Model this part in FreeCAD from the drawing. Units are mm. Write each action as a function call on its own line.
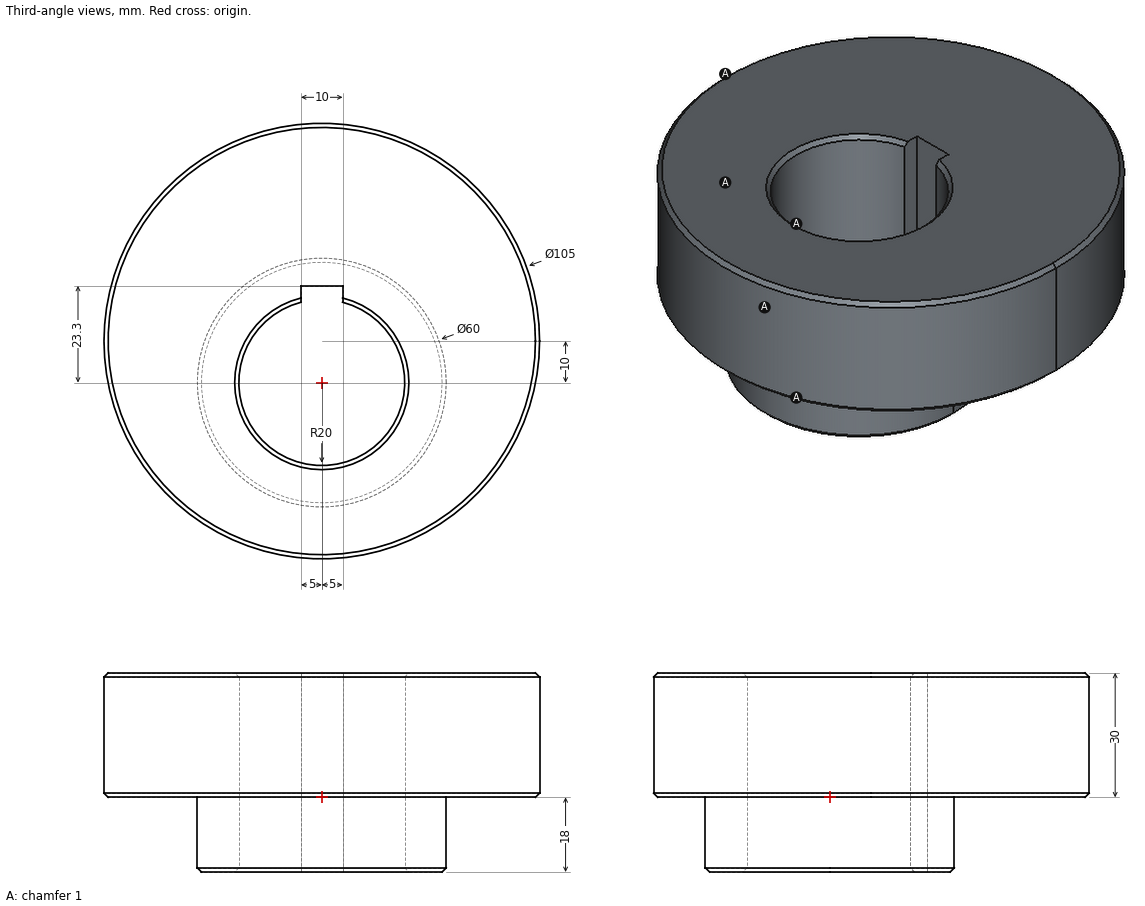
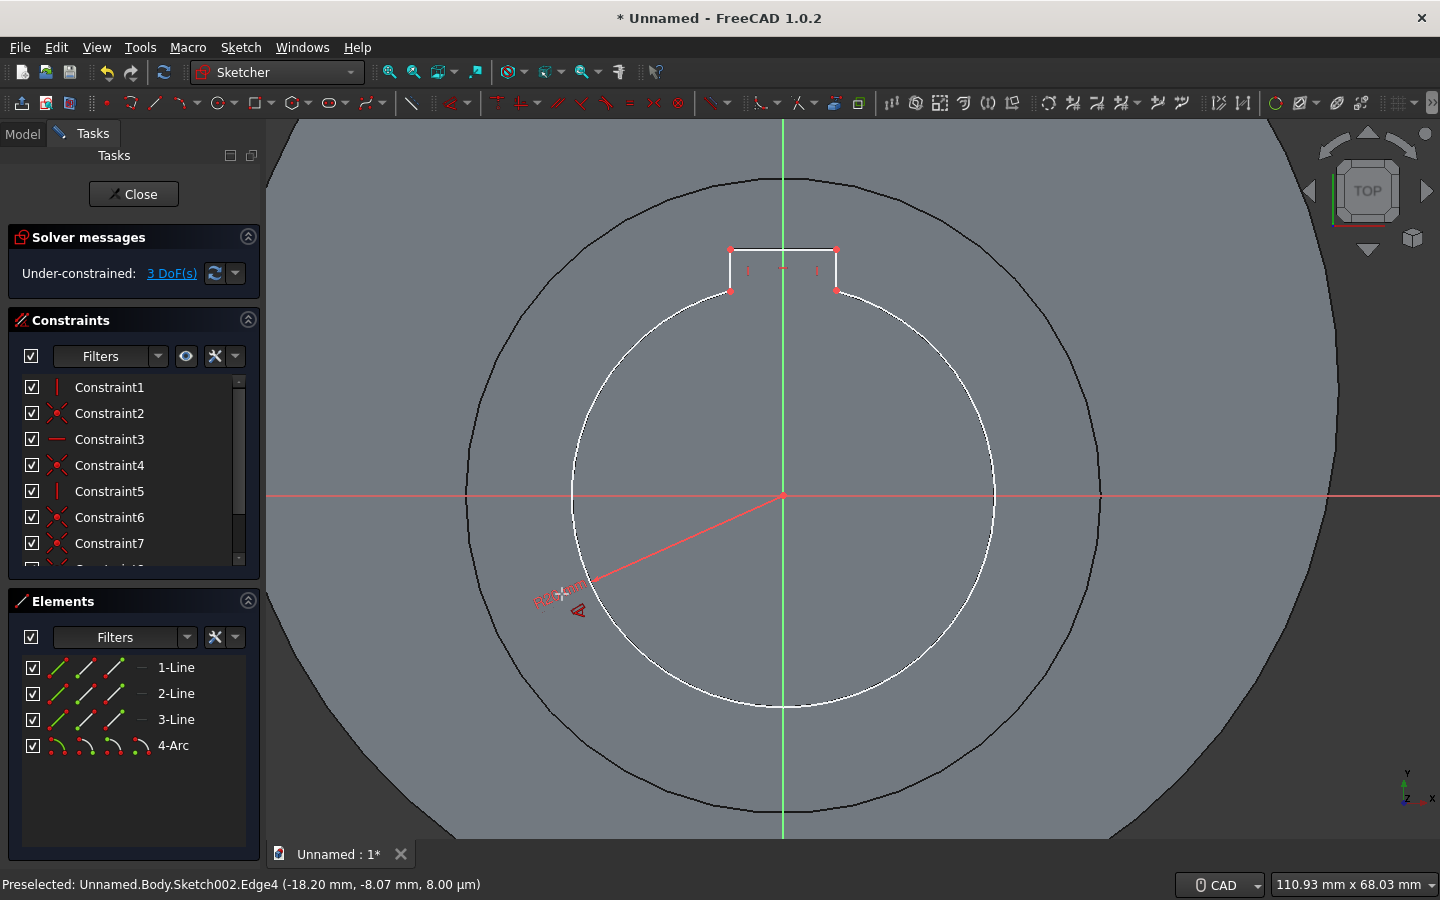
click(804, 250)
click(759, 216)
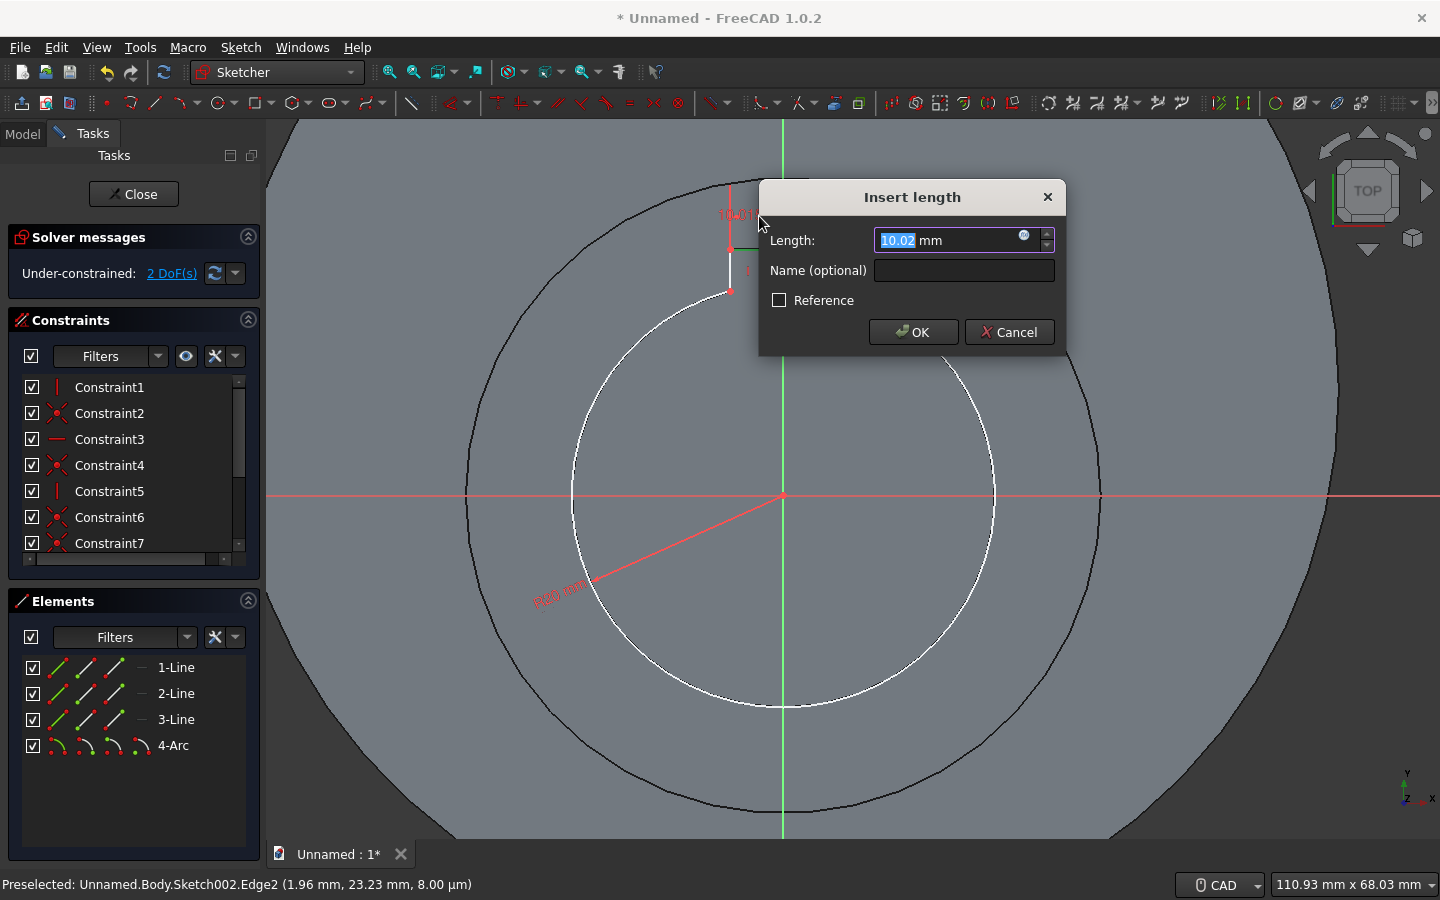
text(10)
key(Return)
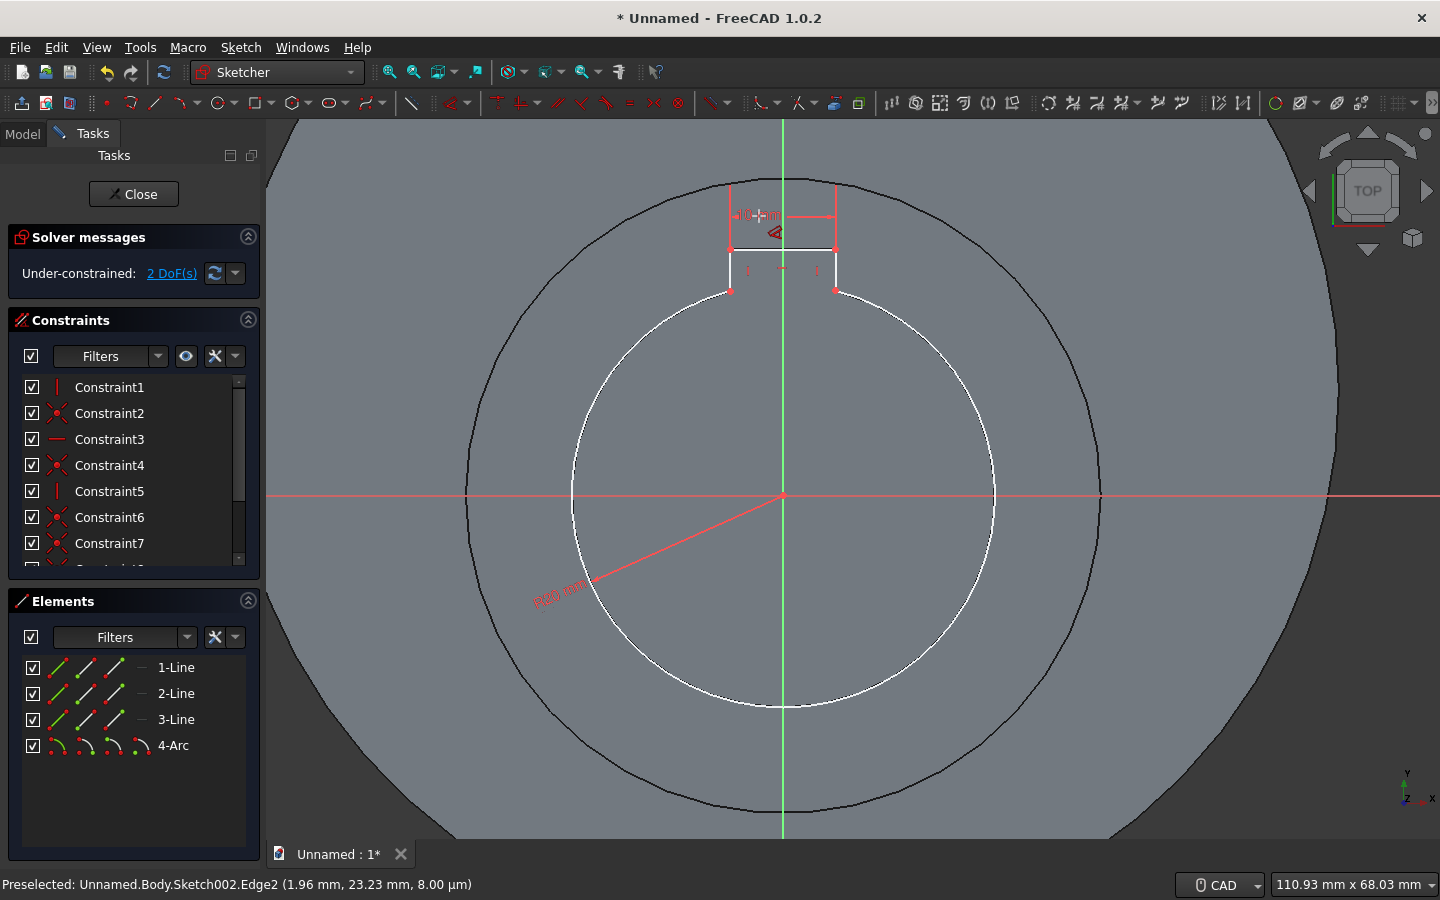
click(836, 291)
click(810, 530)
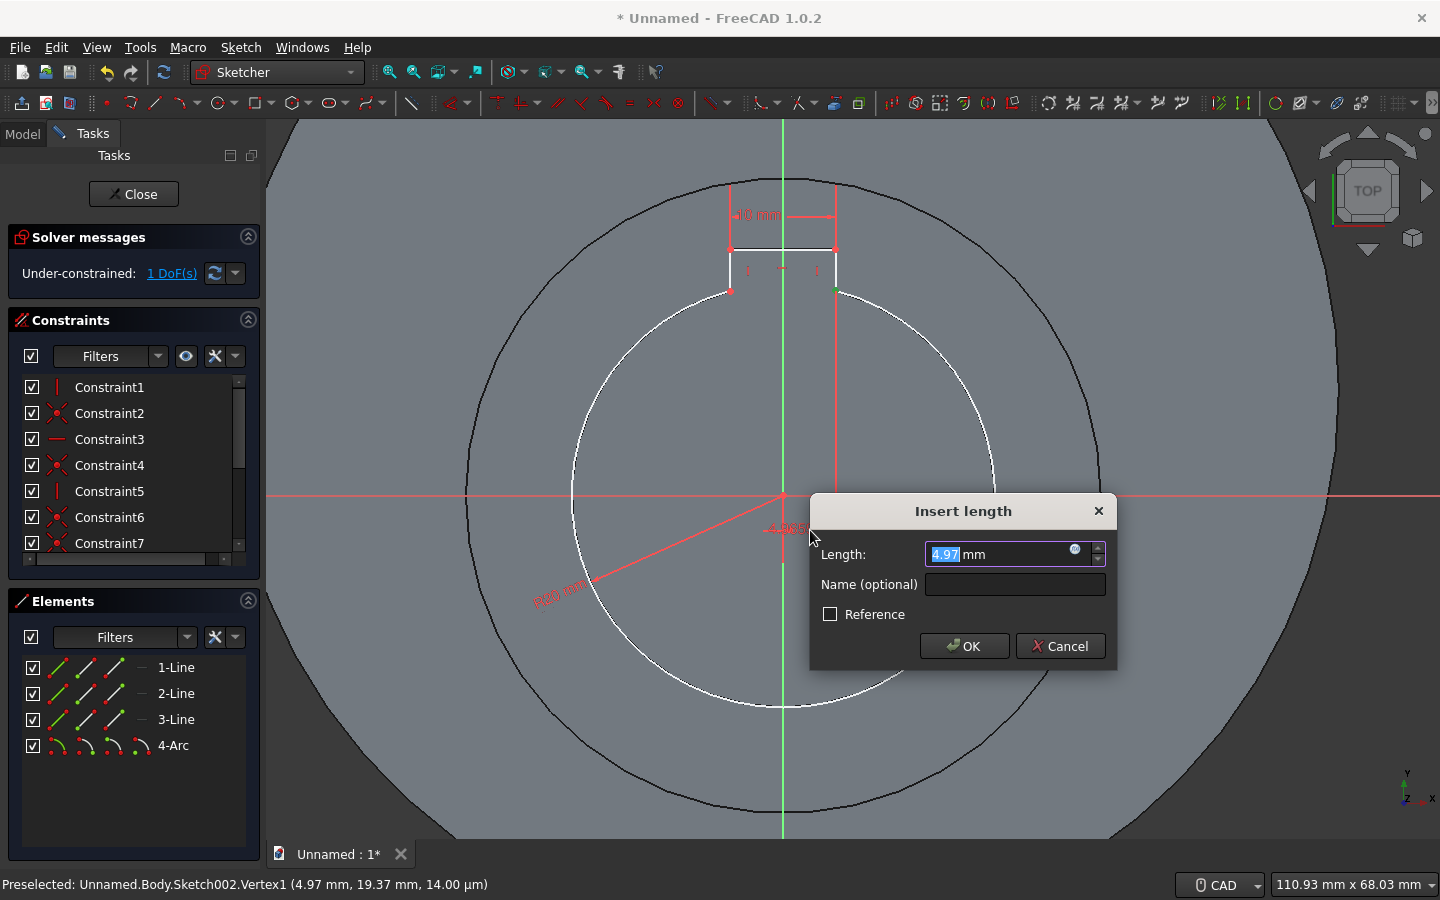
text(5)
key(Return)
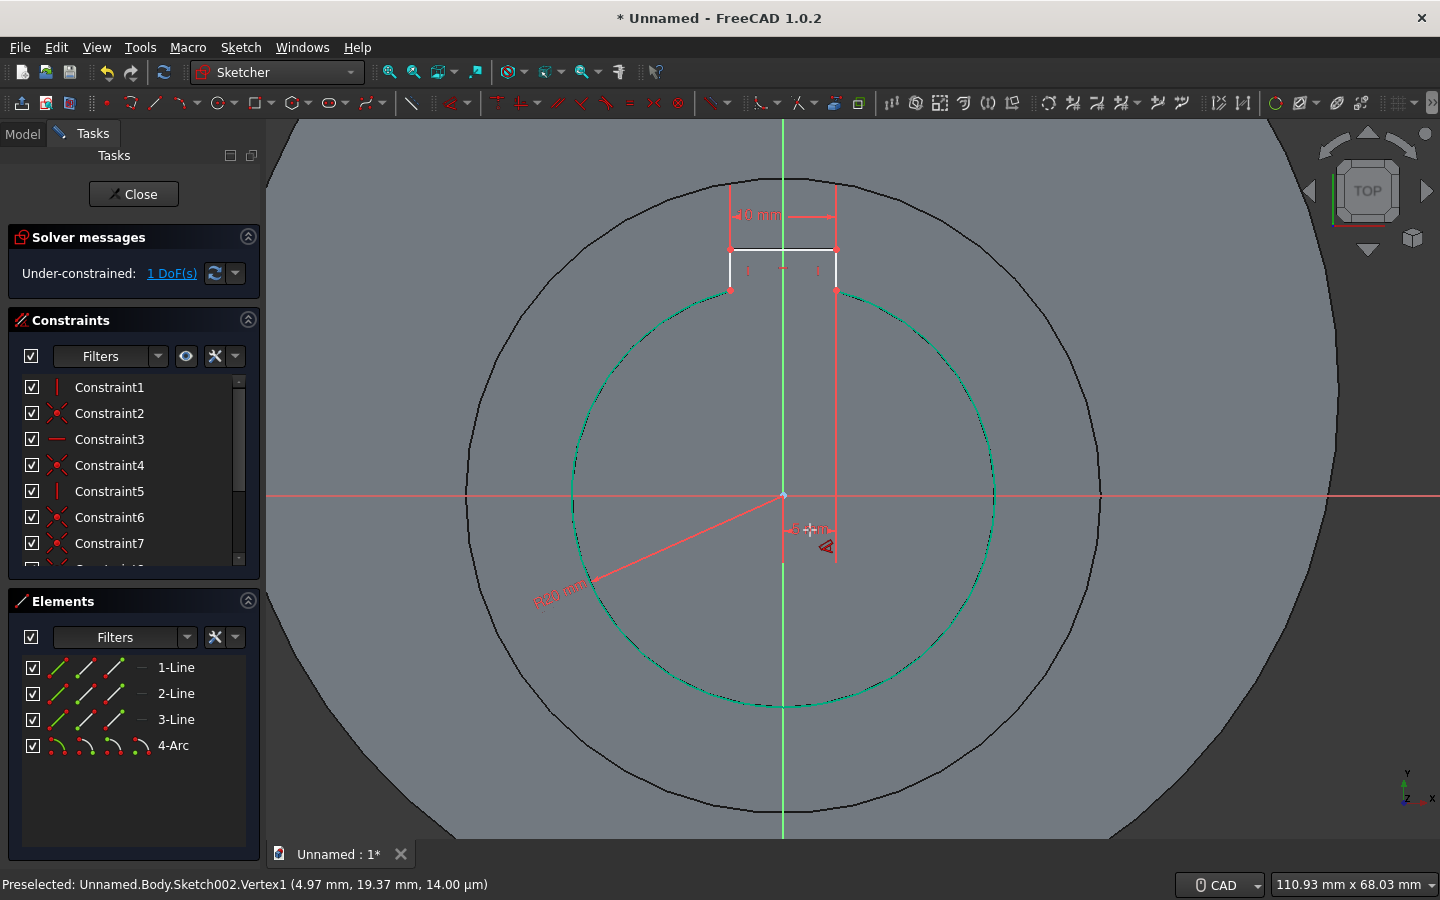
click(836, 250)
click(870, 373)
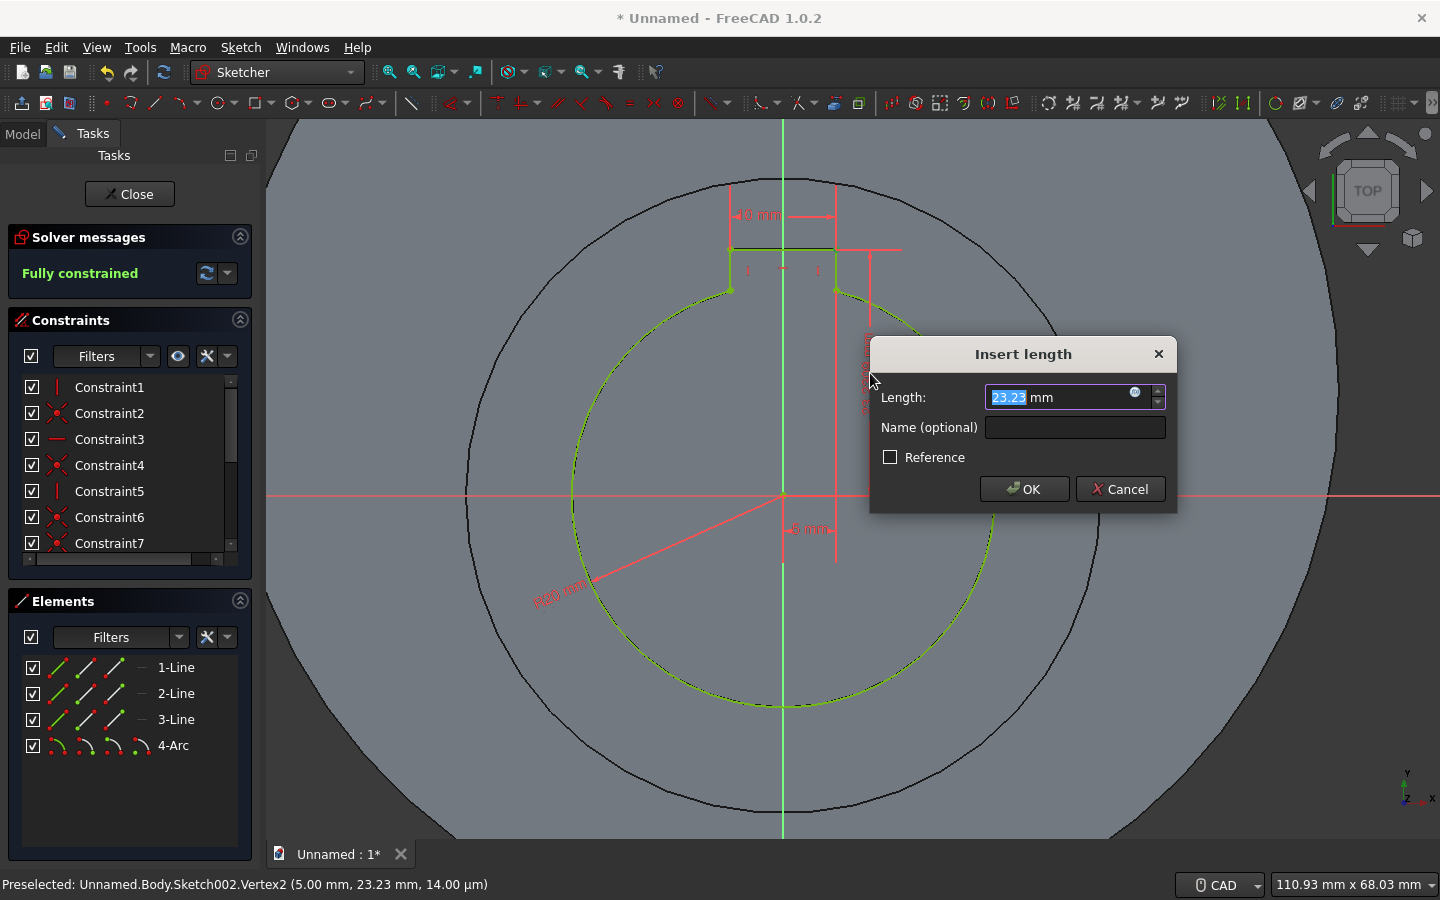
text(23.3)
key(Return)
key(Escape)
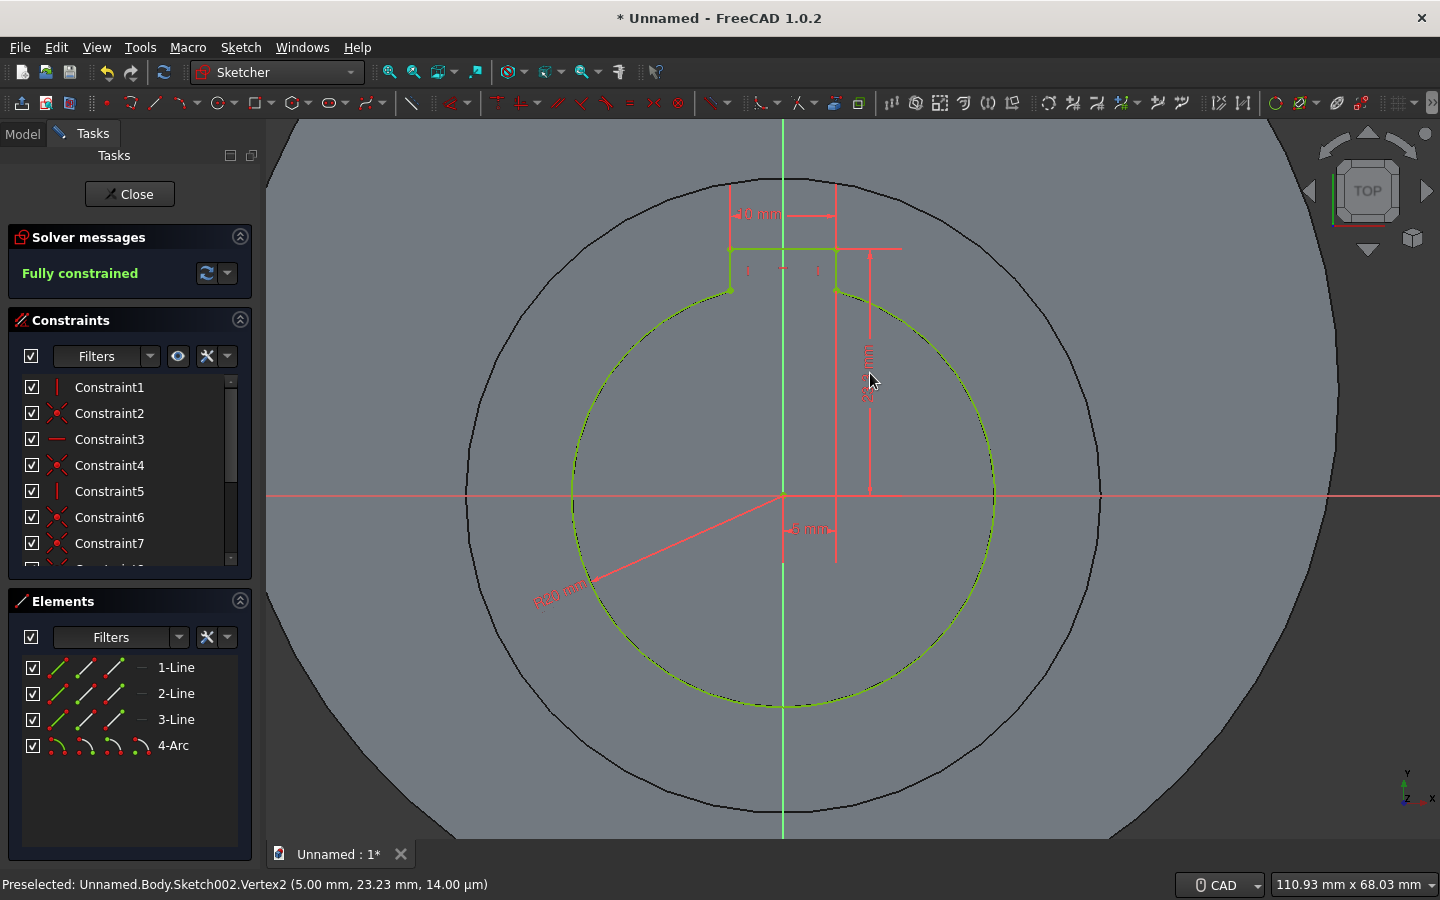
click(130, 194)